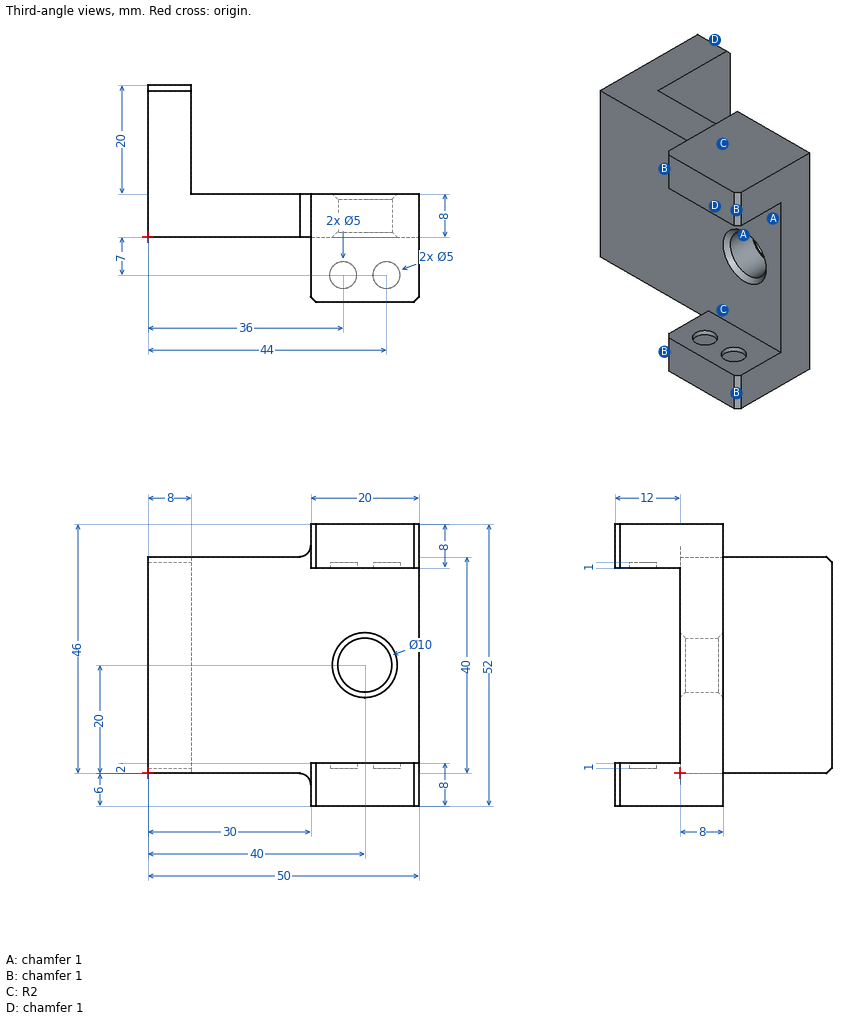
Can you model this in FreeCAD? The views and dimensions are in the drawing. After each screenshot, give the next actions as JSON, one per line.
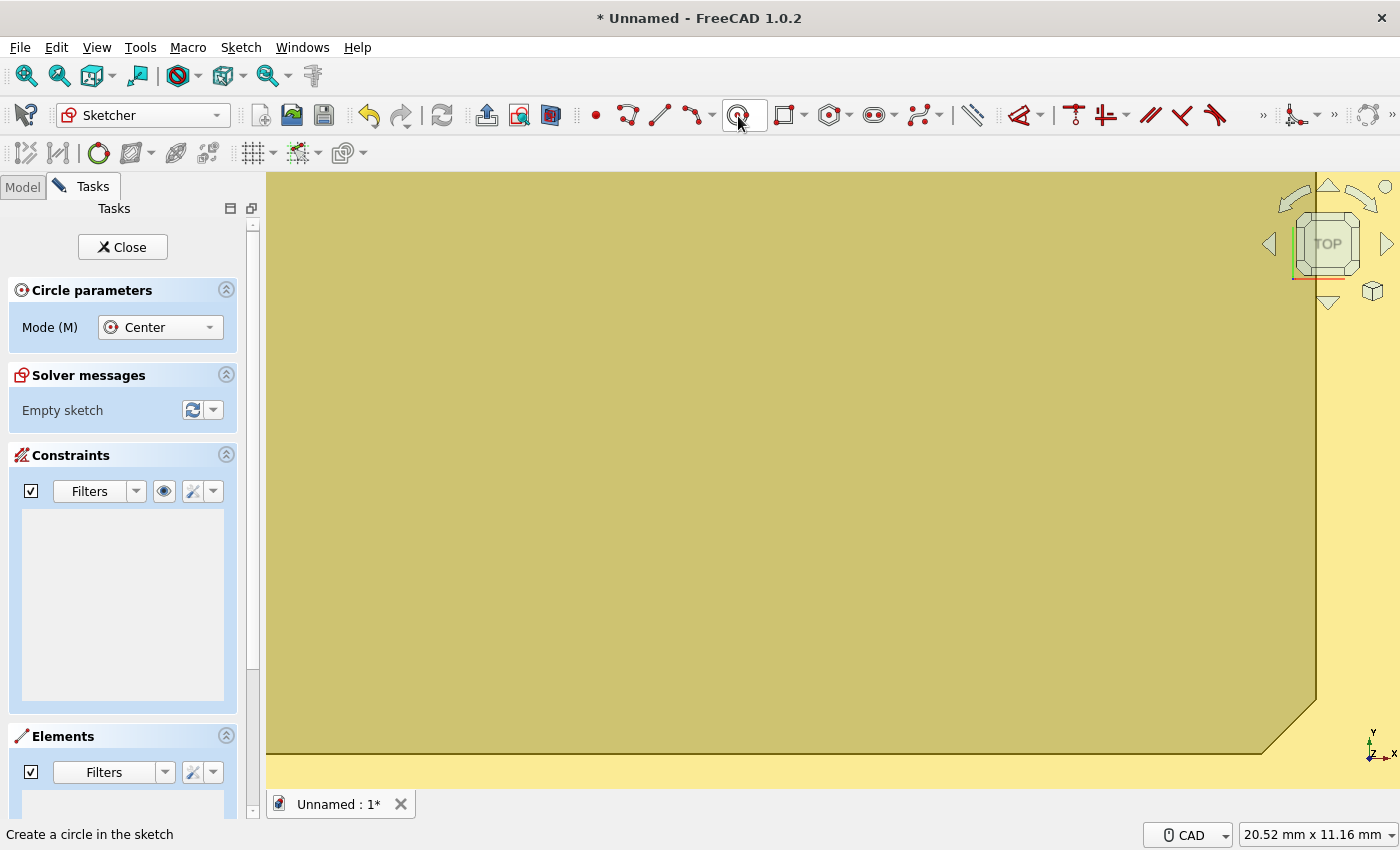
{"action": "left_click", "coordinate": [985, 478]}
{"action": "mouse_move", "coordinate": [1082, 380]}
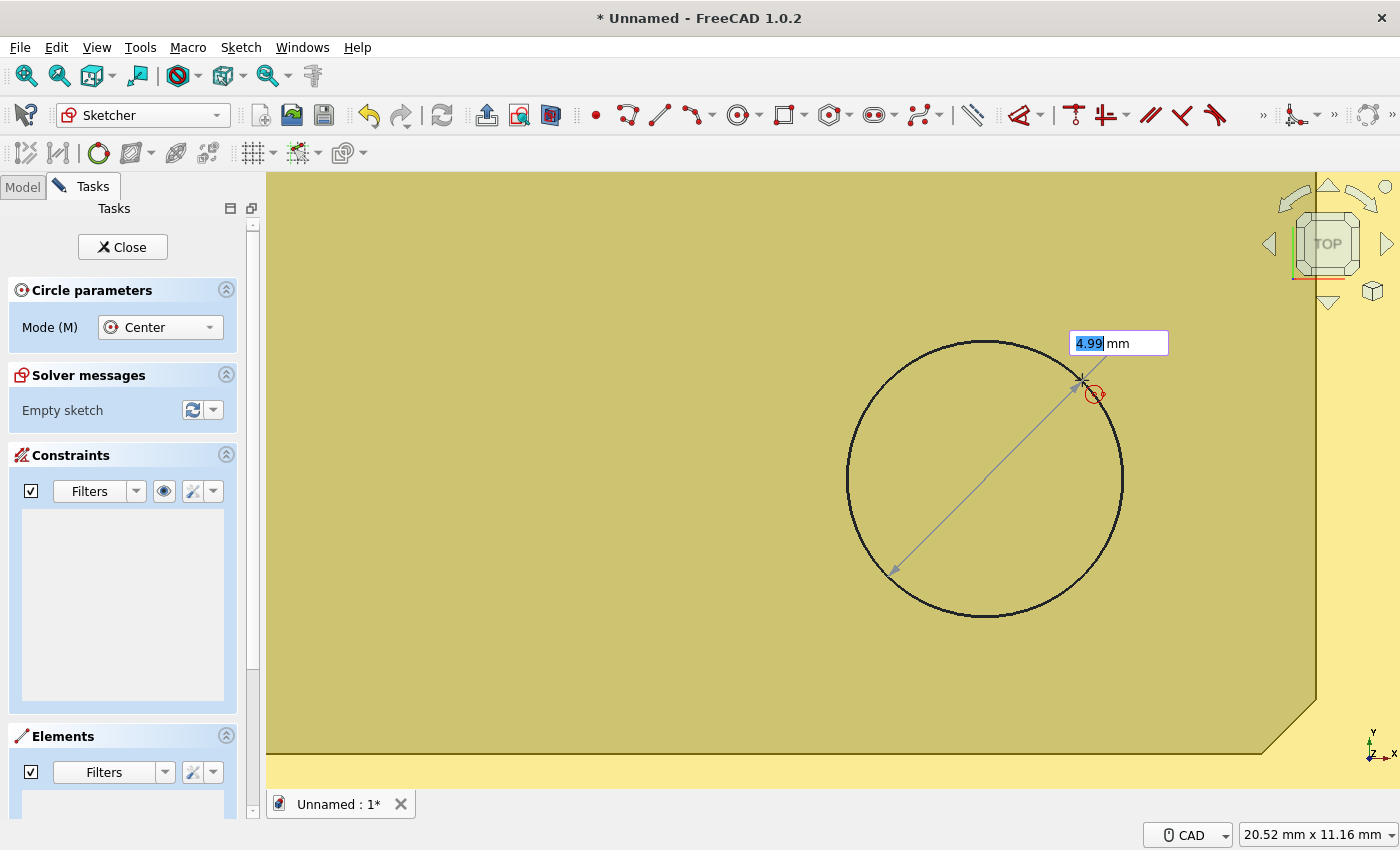
{"action": "type", "text": "5"}
{"action": "key", "text": "Return"}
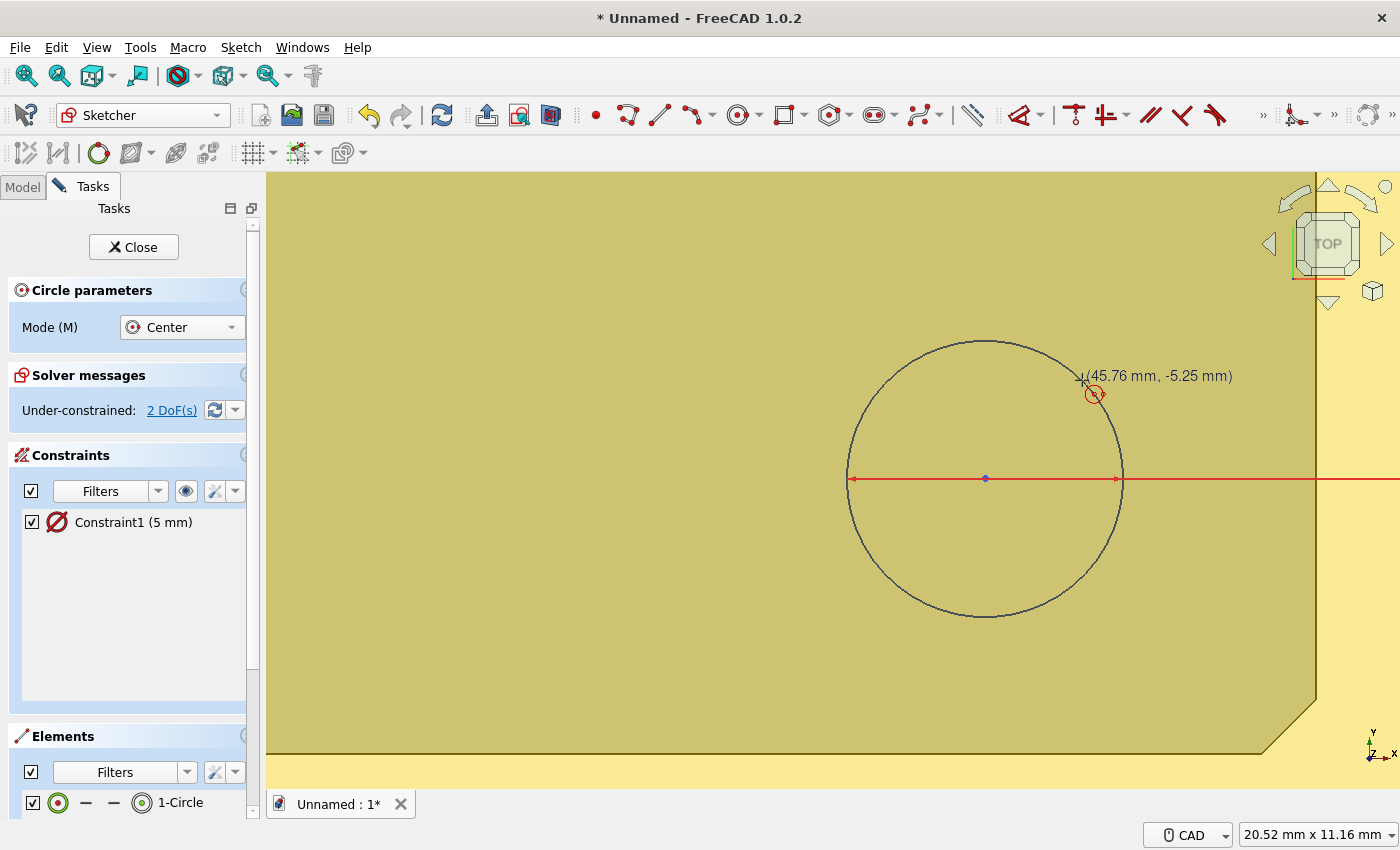
{"action": "left_click", "coordinate": [543, 478]}
{"action": "mouse_move", "coordinate": [640, 380]}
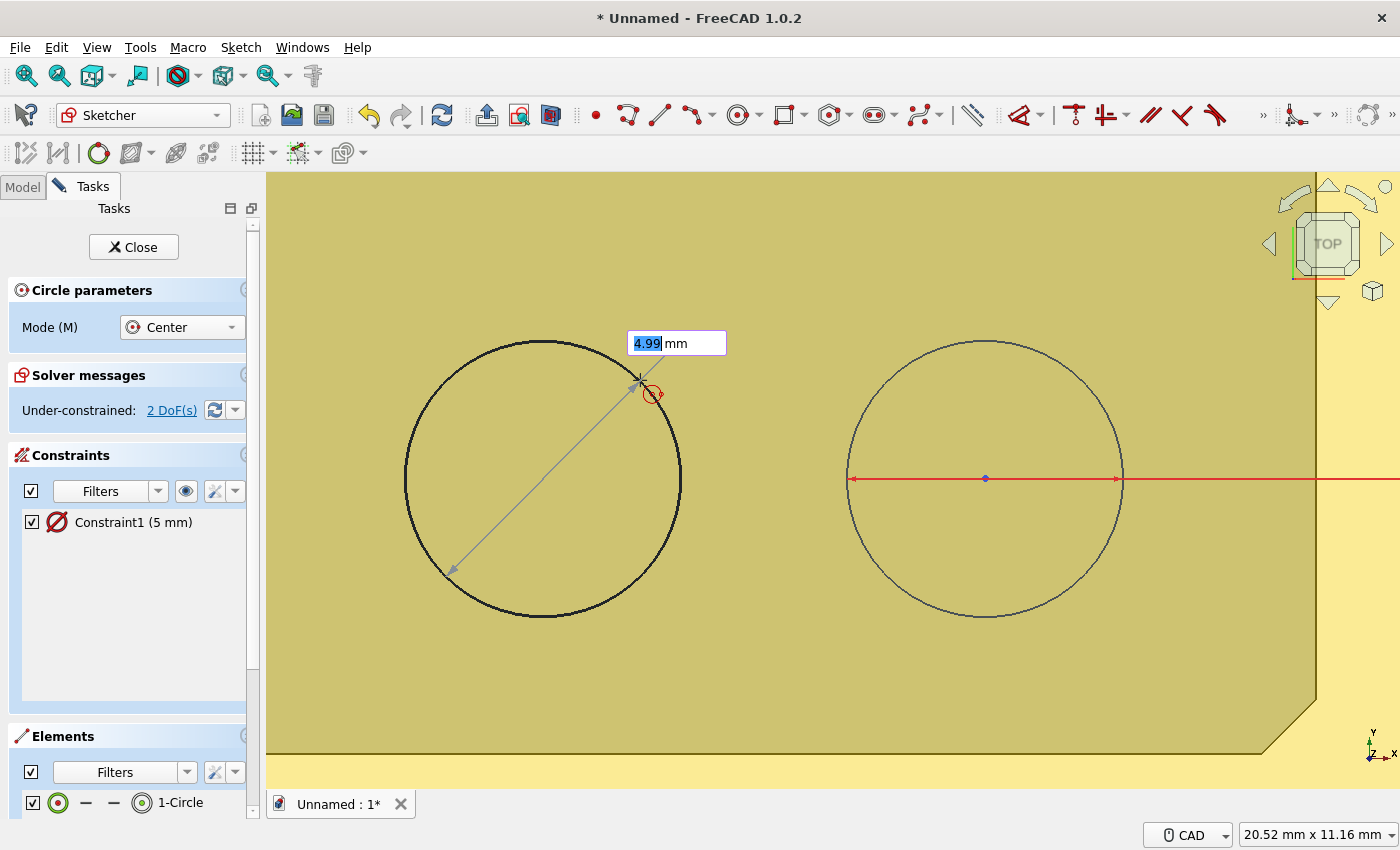
{"action": "type", "text": "5"}
{"action": "key", "text": "Return"}
{"action": "key", "text": "Escape"}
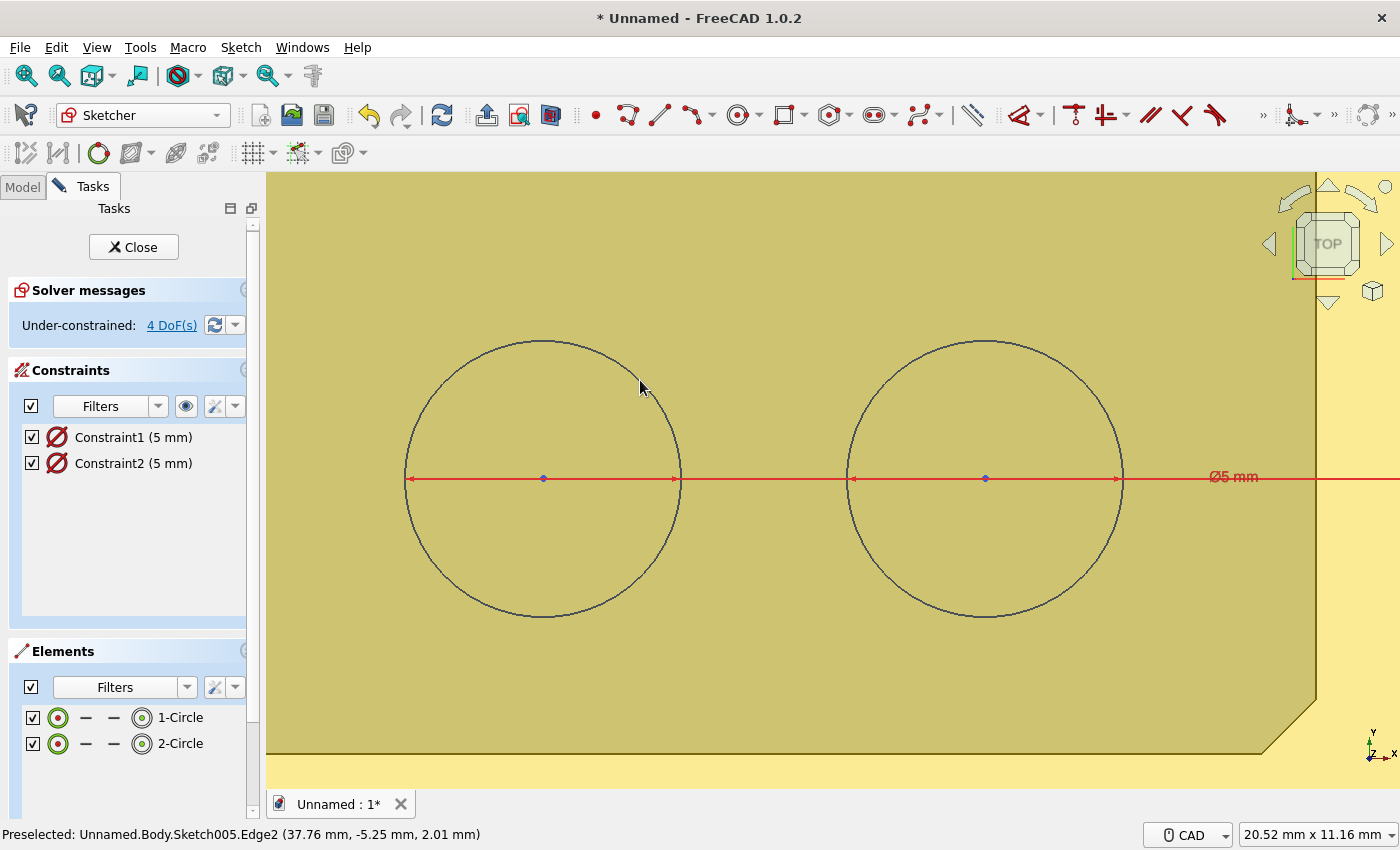
{"action": "left_click", "coordinate": [985, 479]}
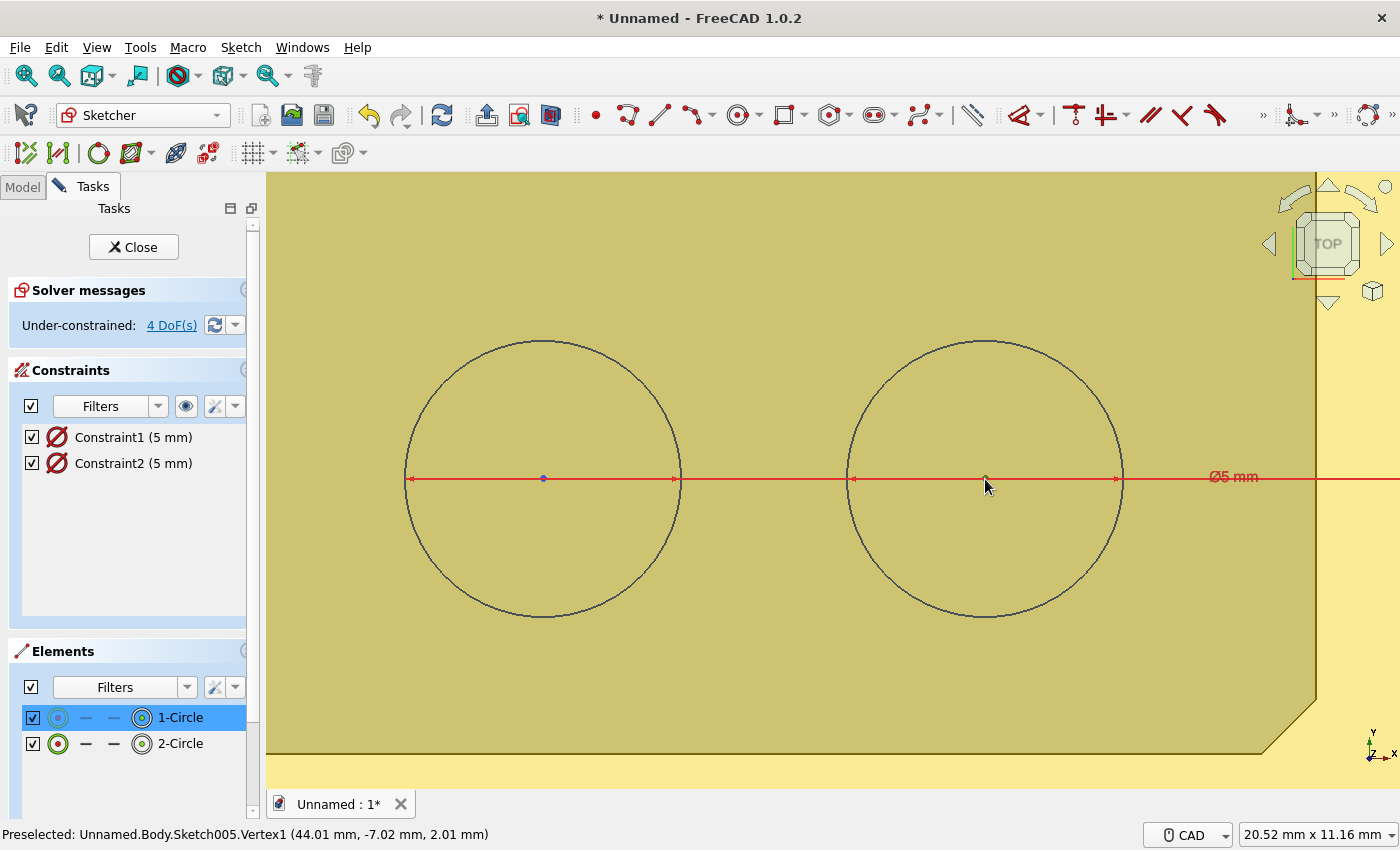
{"action": "left_click", "coordinate": [543, 479]}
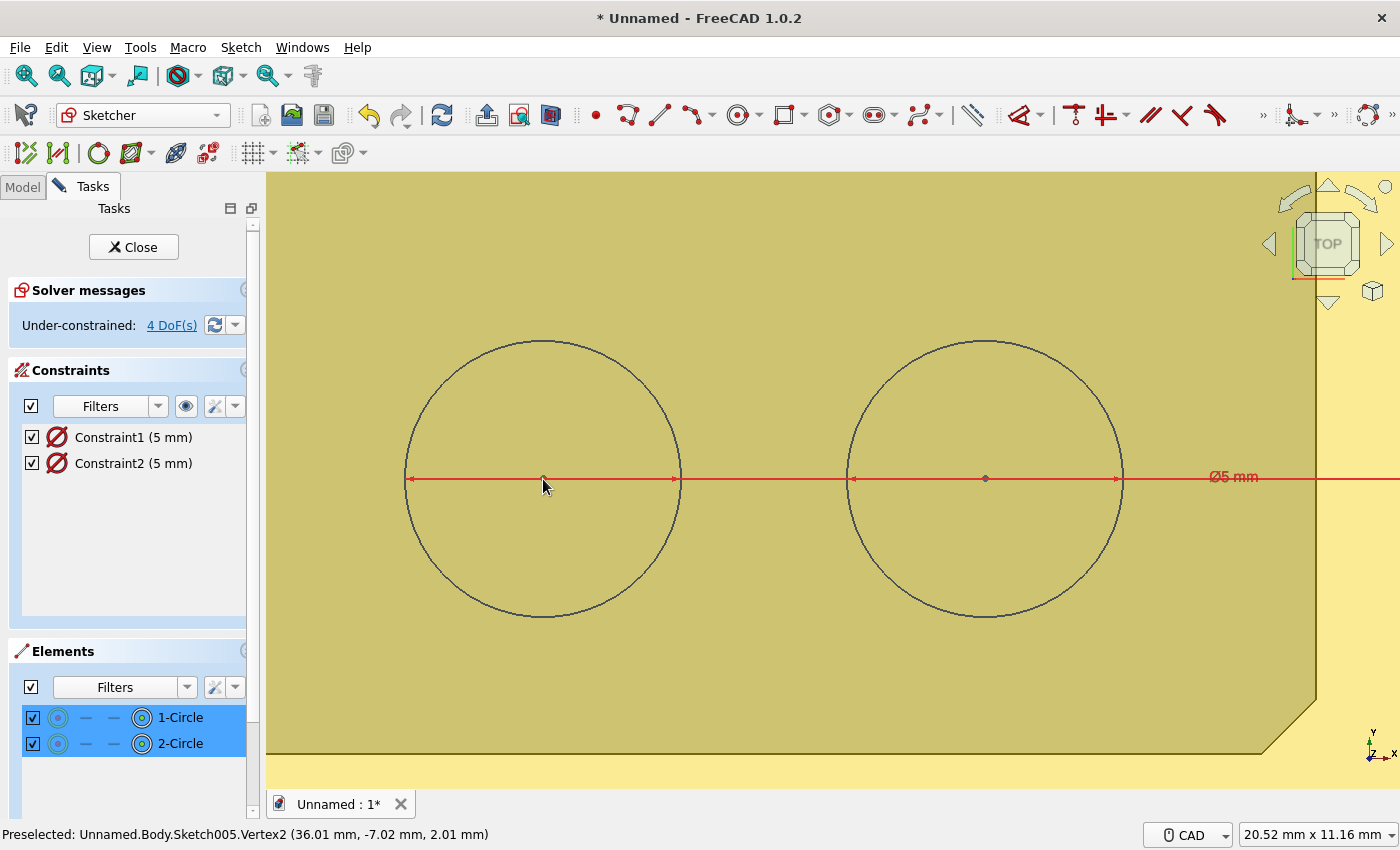
{"action": "key", "text": "h"}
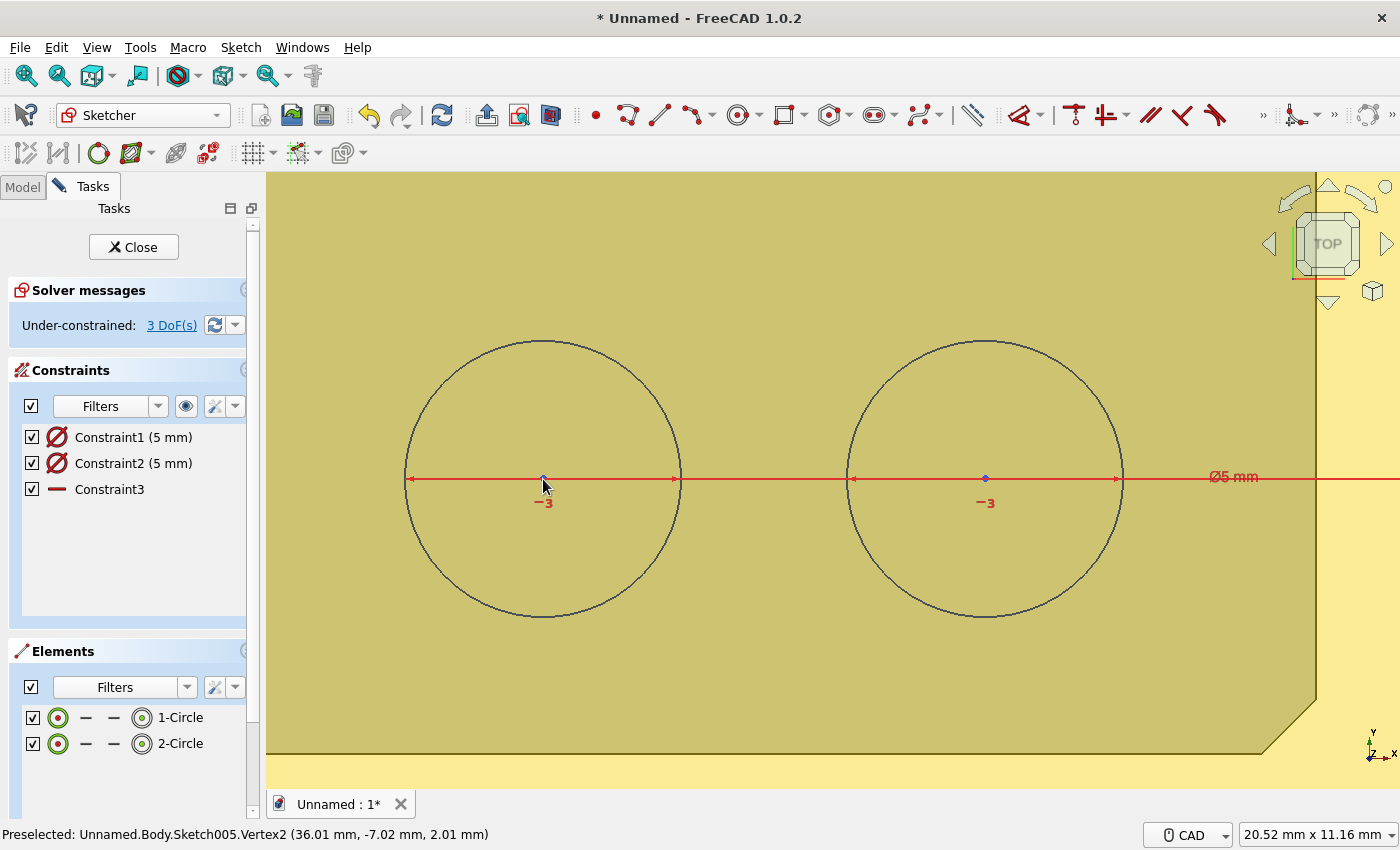
{"action": "left_click", "coordinate": [1020, 116]}